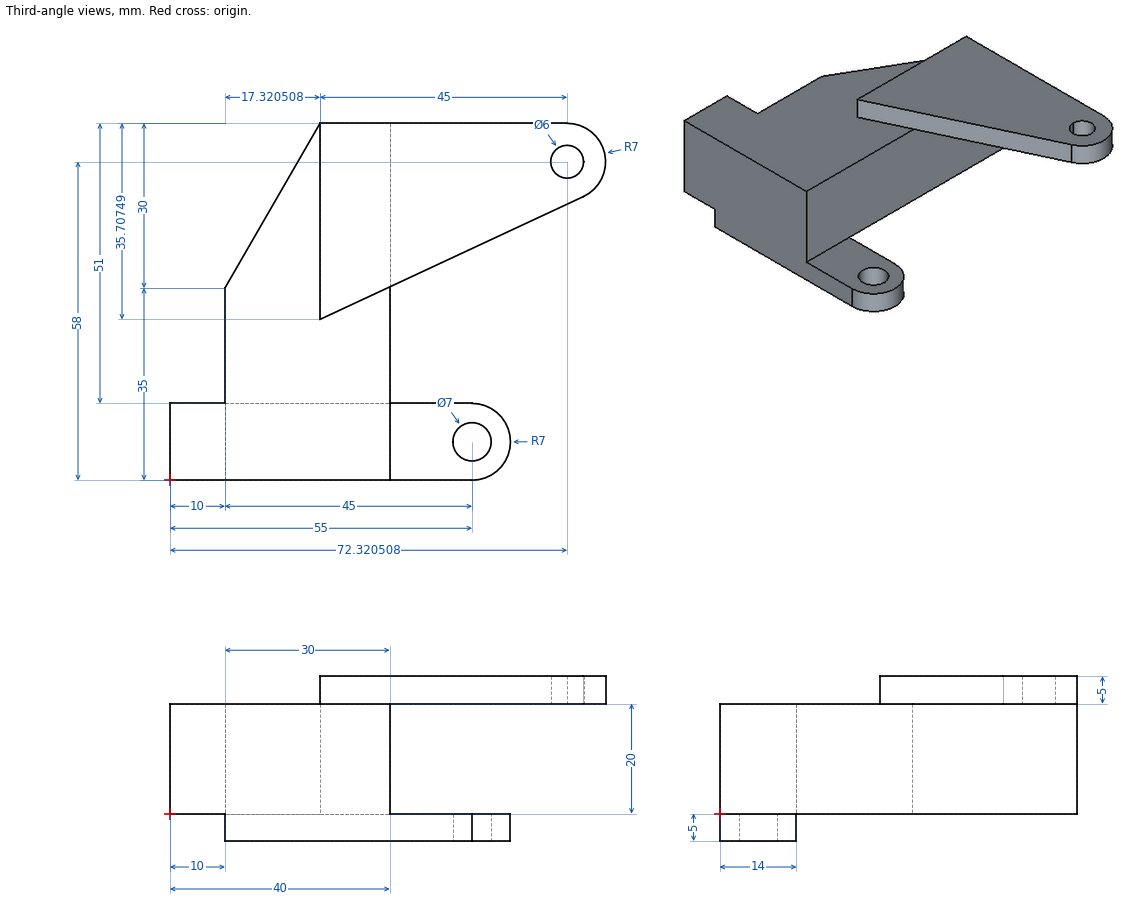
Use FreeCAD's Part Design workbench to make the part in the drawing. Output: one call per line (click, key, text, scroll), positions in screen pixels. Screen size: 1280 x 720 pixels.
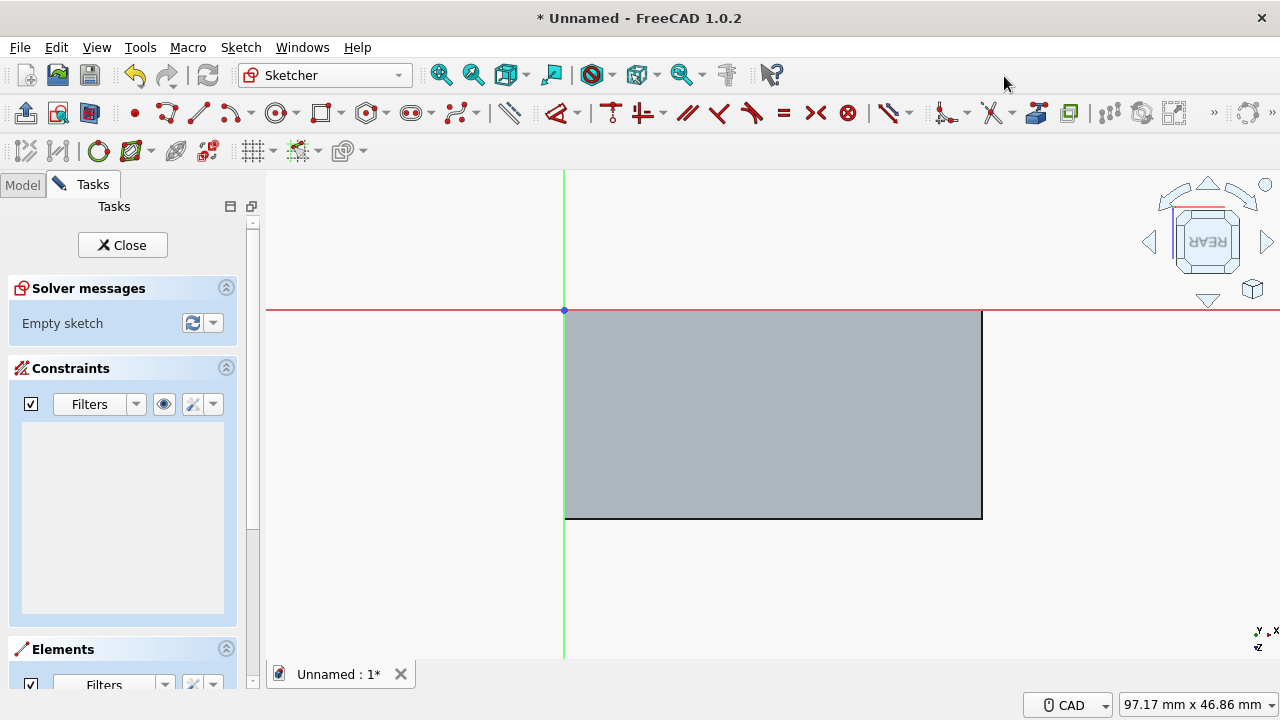
scroll(912, 414, up, 2)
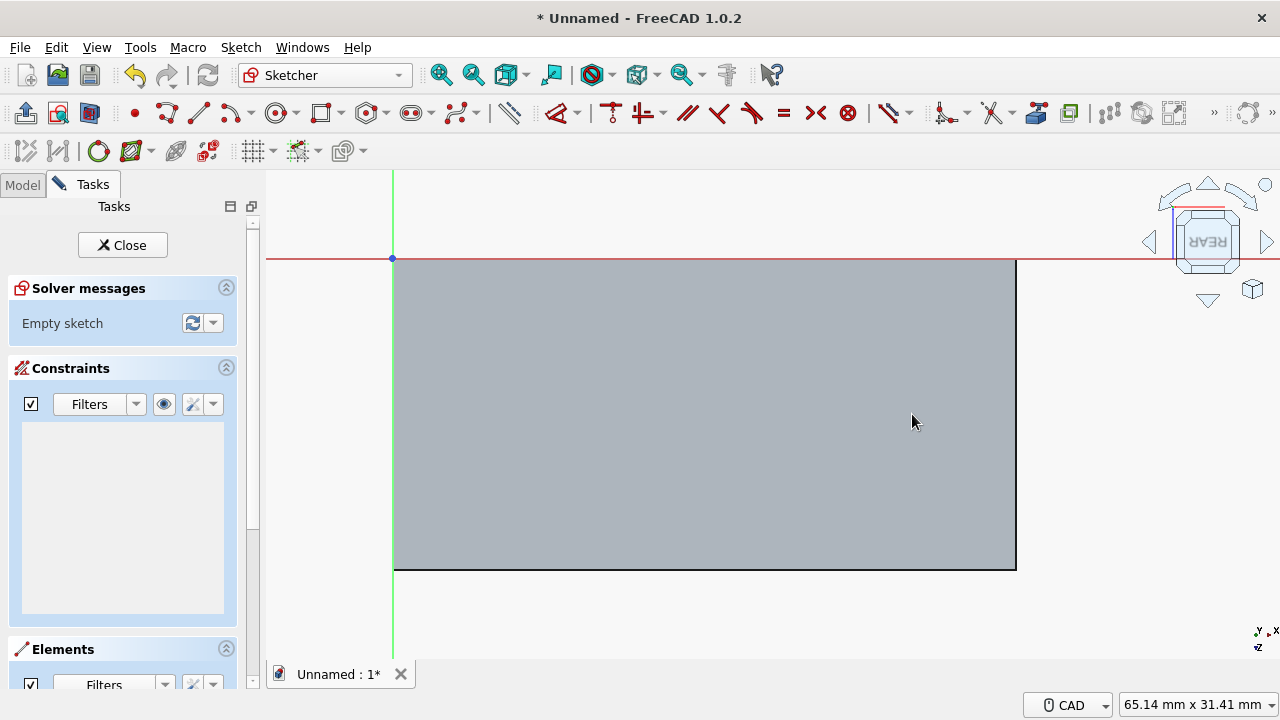
key(g)
key(r)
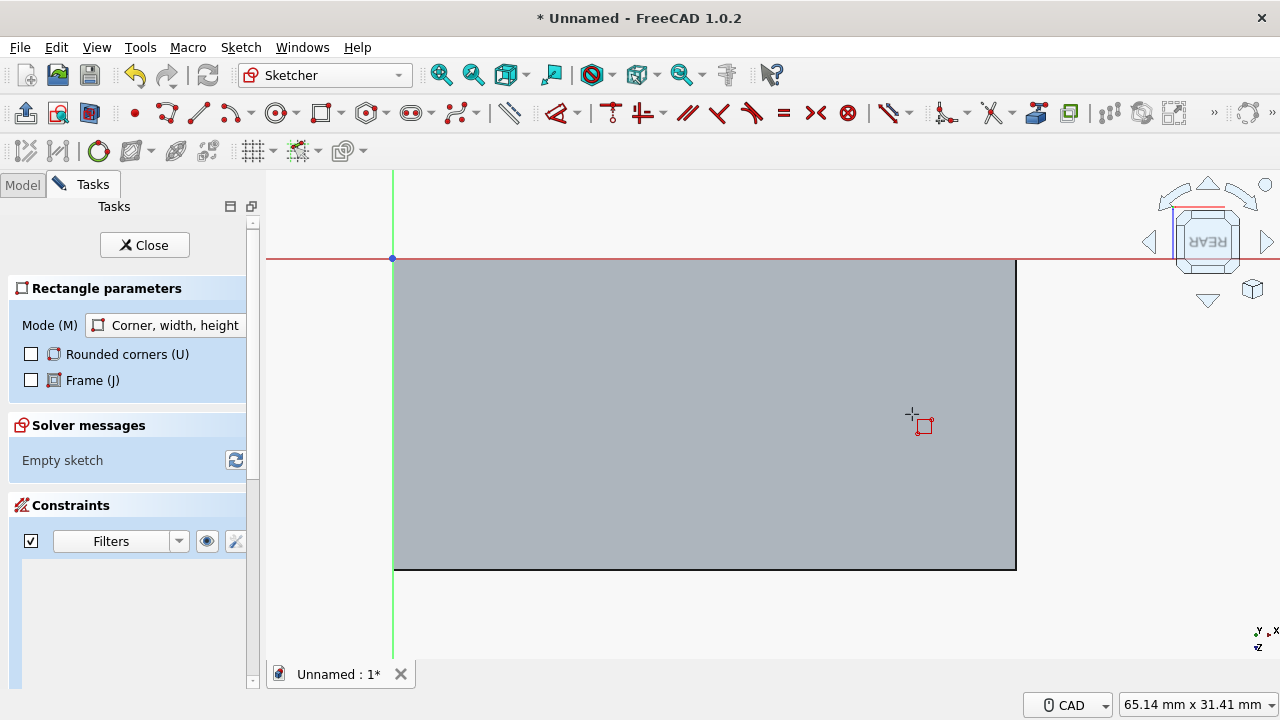
click(549, 259)
click(1016, 570)
key(Escape)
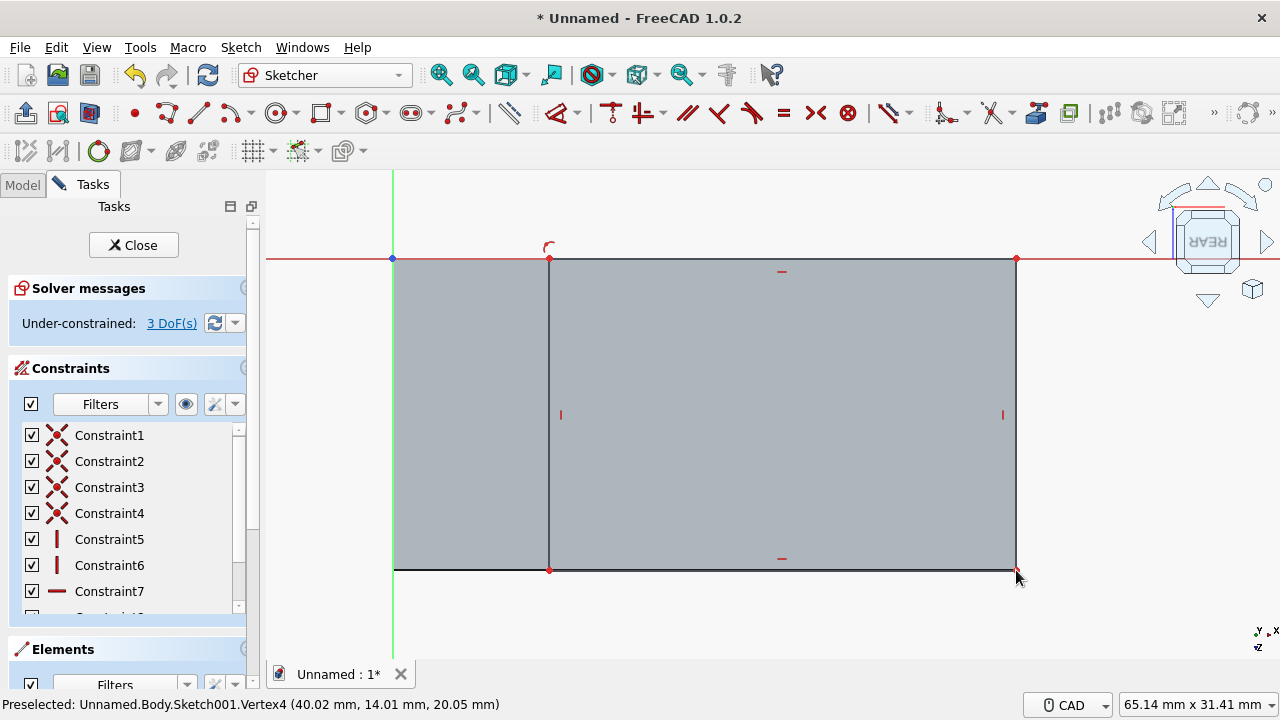
click(556, 114)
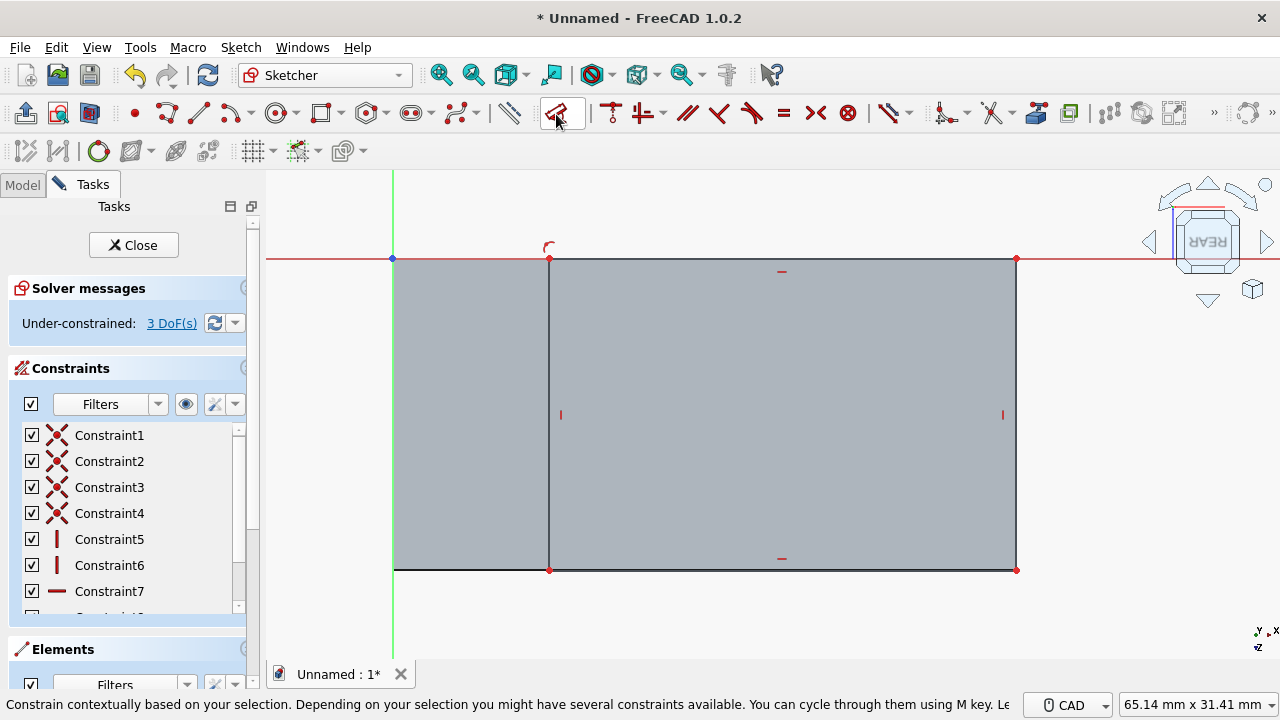
click(549, 352)
click(515, 415)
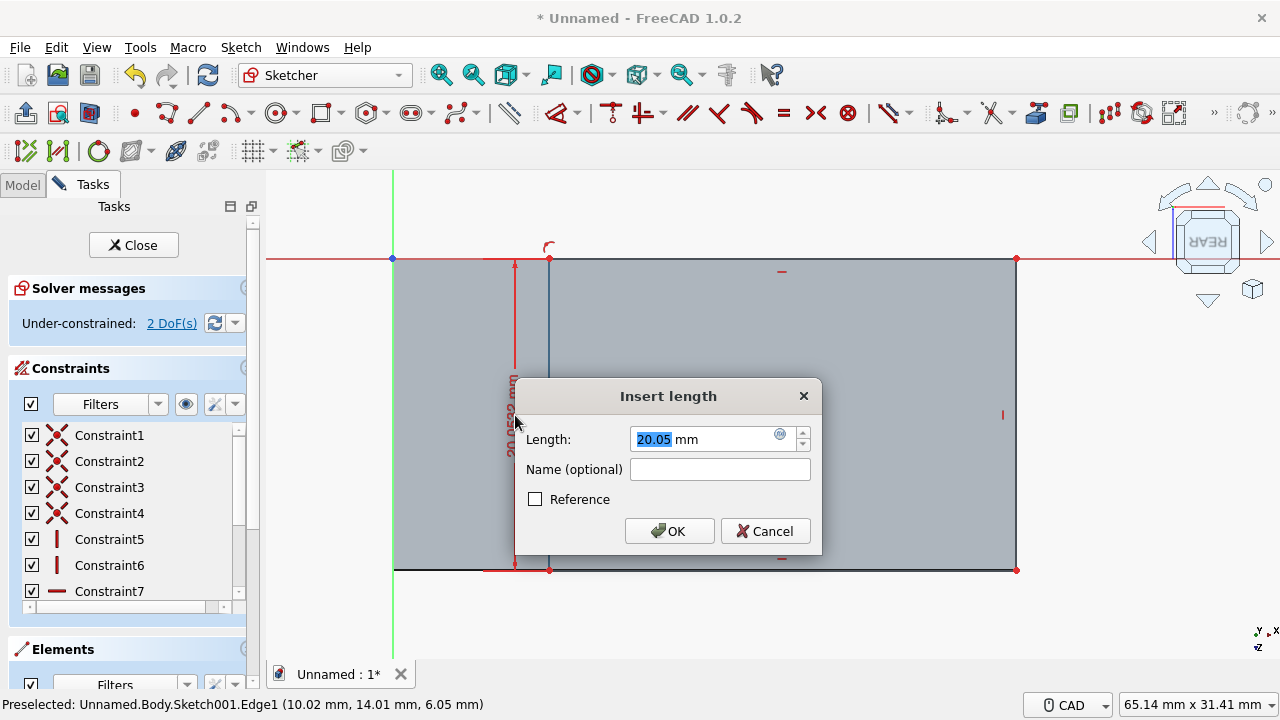
text(20)
key(Return)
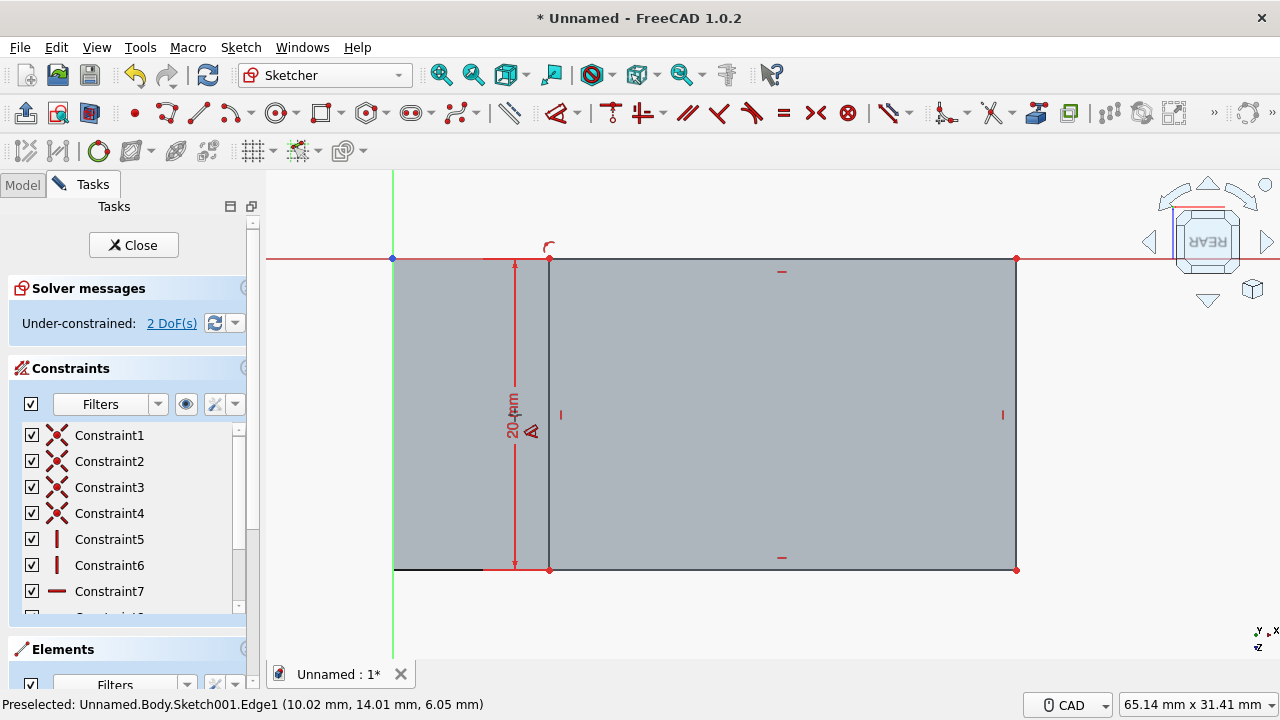
click(689, 570)
click(782, 604)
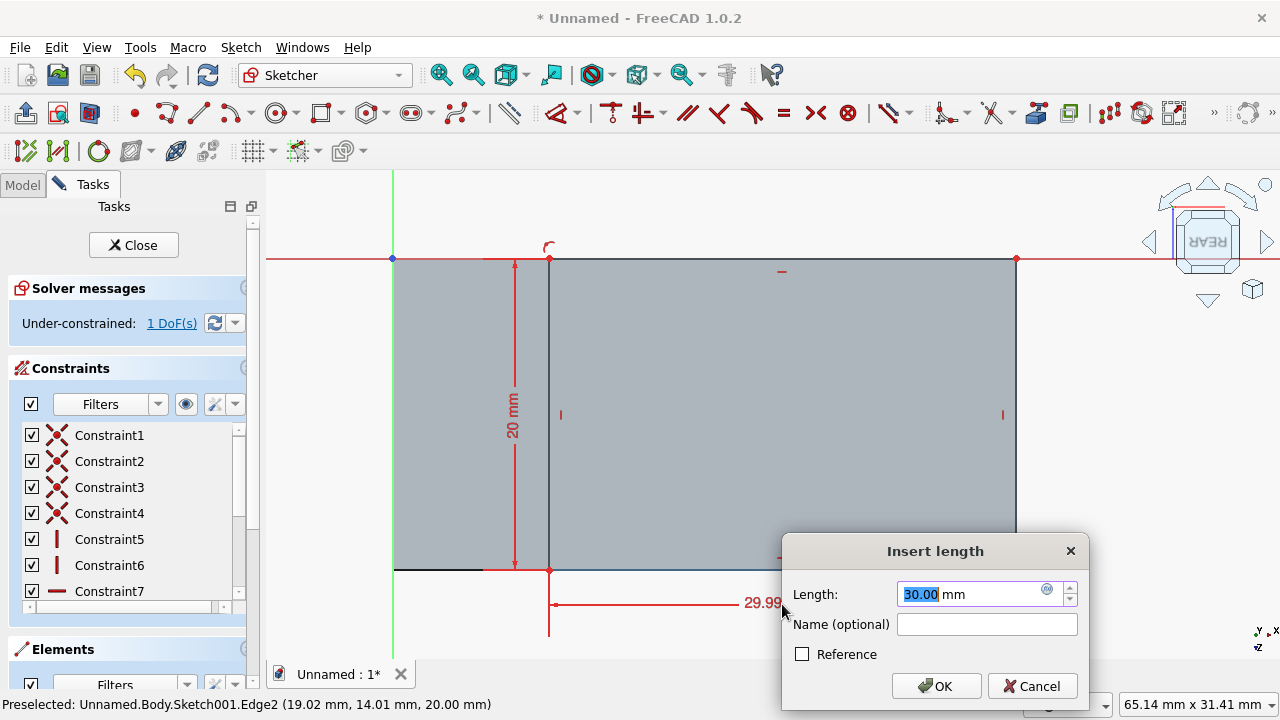
text(30)
key(Return)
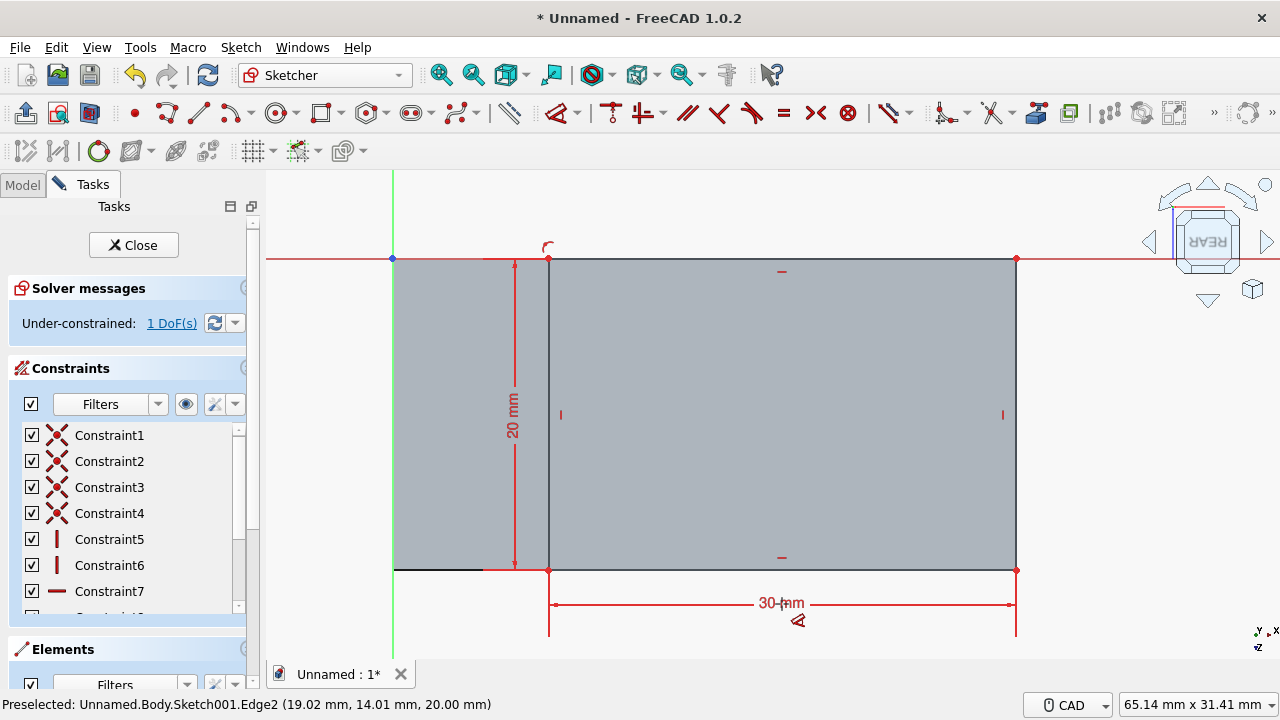
click(549, 259)
click(471, 225)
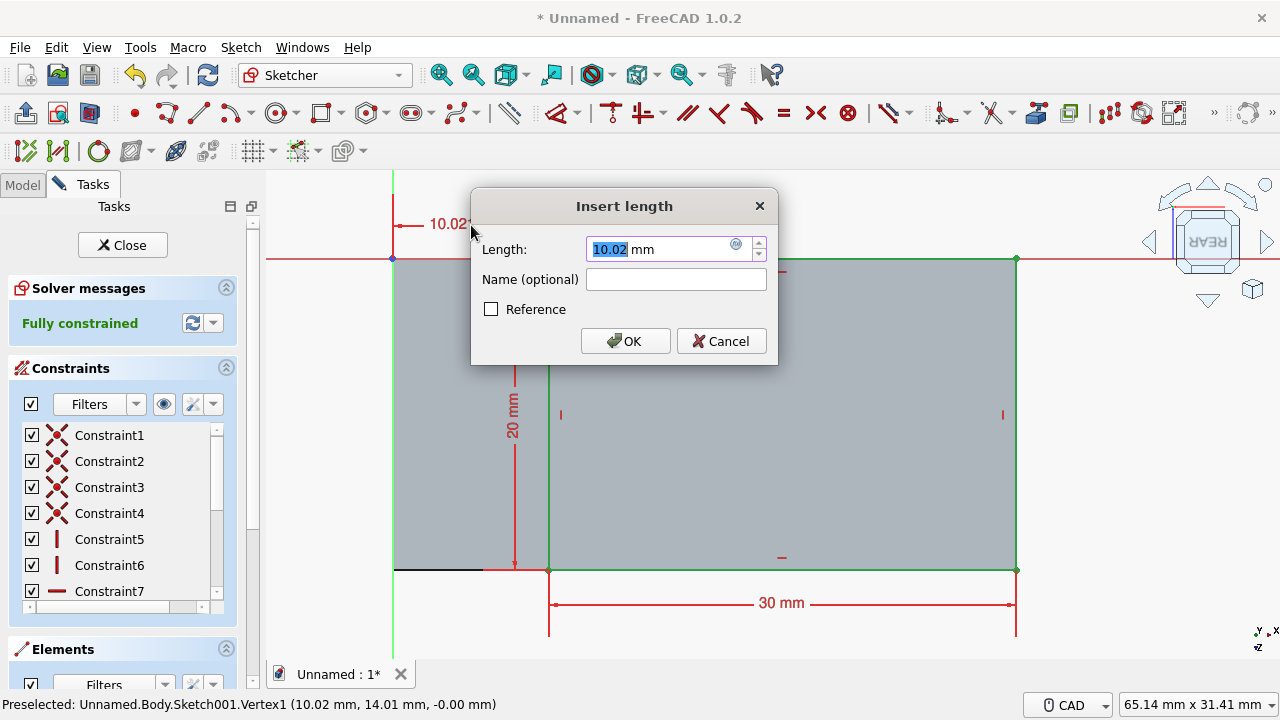
text(10)
key(Return)
key(Escape)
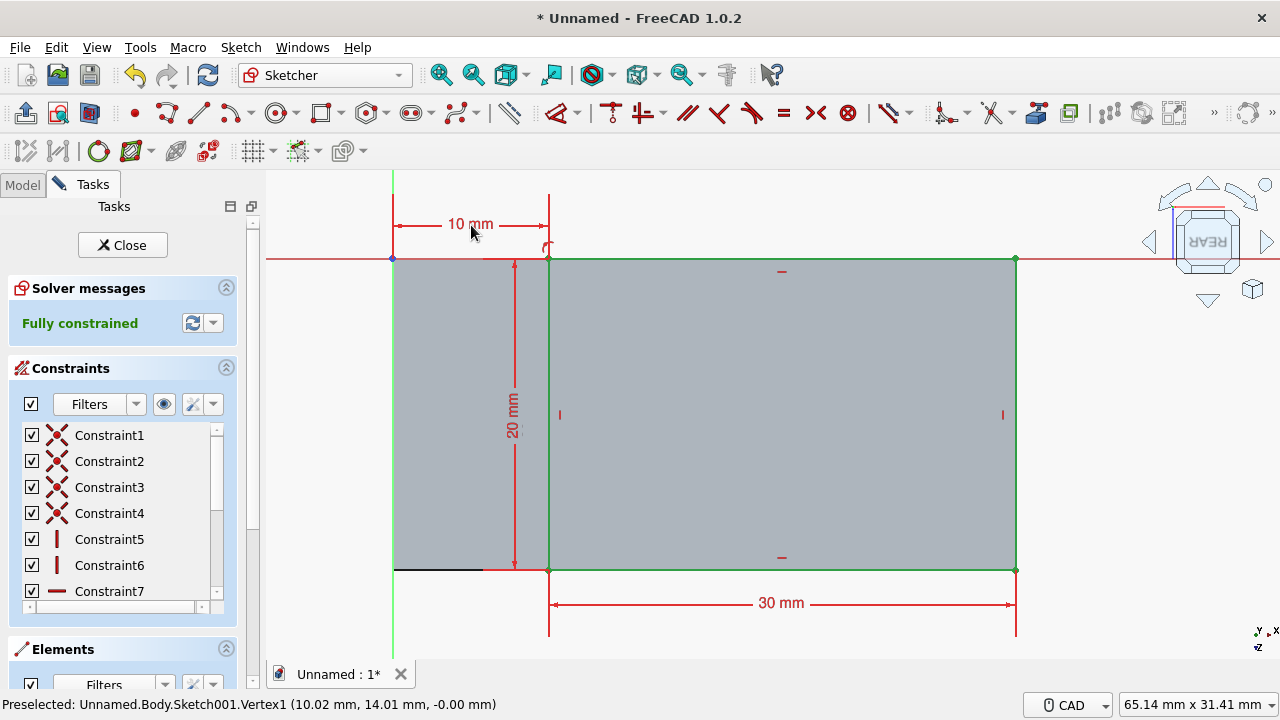
click(123, 245)